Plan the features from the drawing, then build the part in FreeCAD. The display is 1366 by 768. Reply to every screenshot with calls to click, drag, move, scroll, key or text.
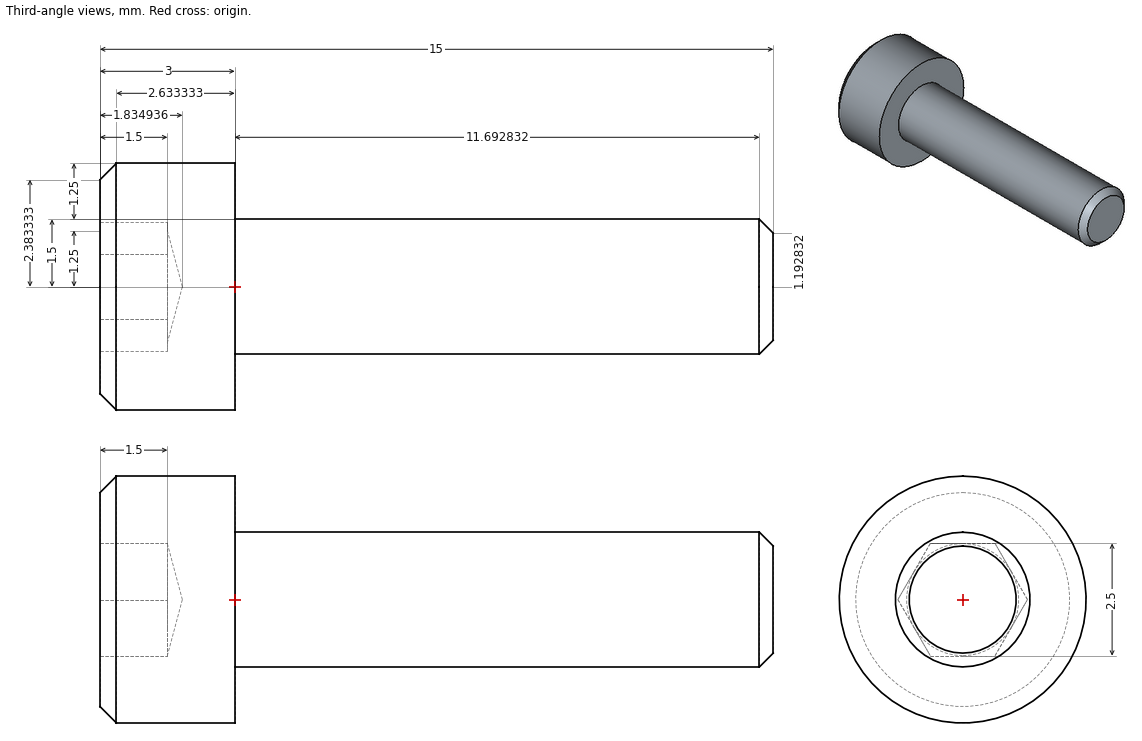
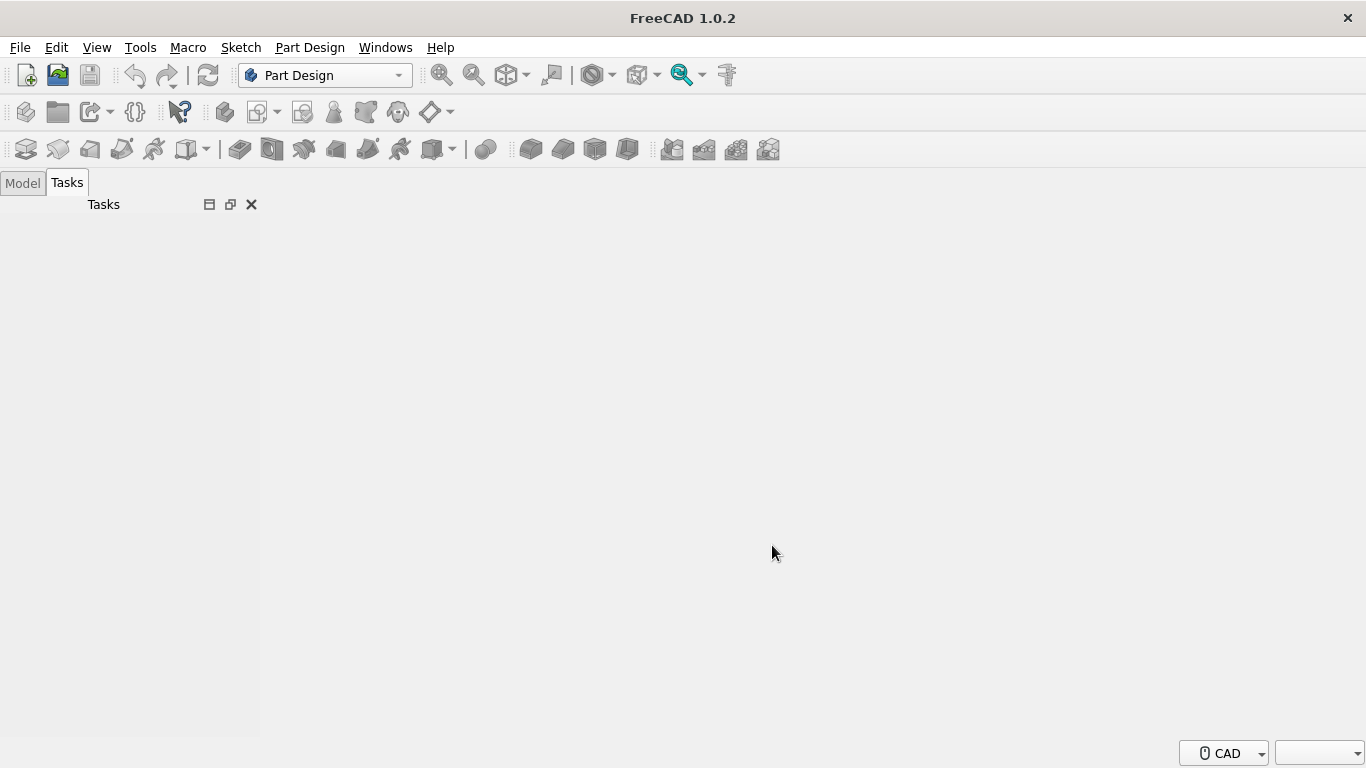
click(26, 76)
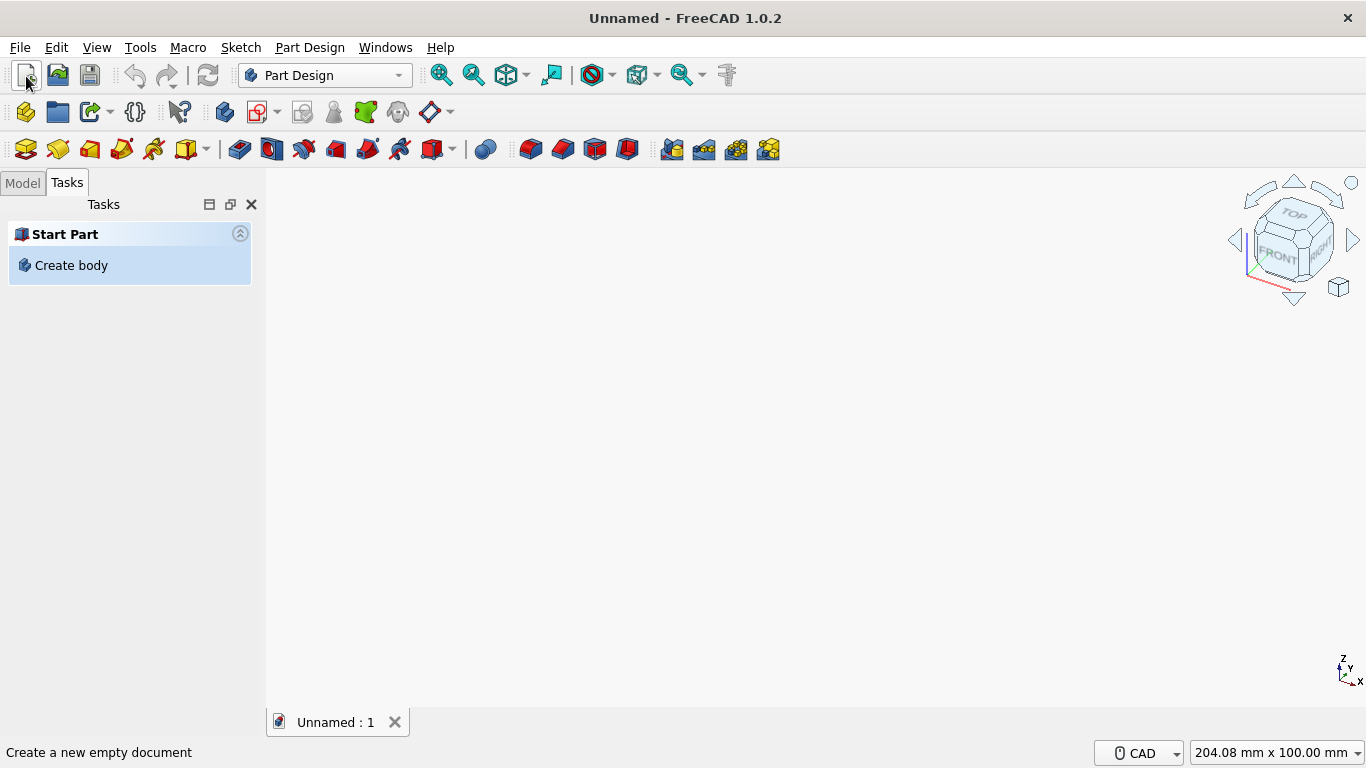
click(258, 112)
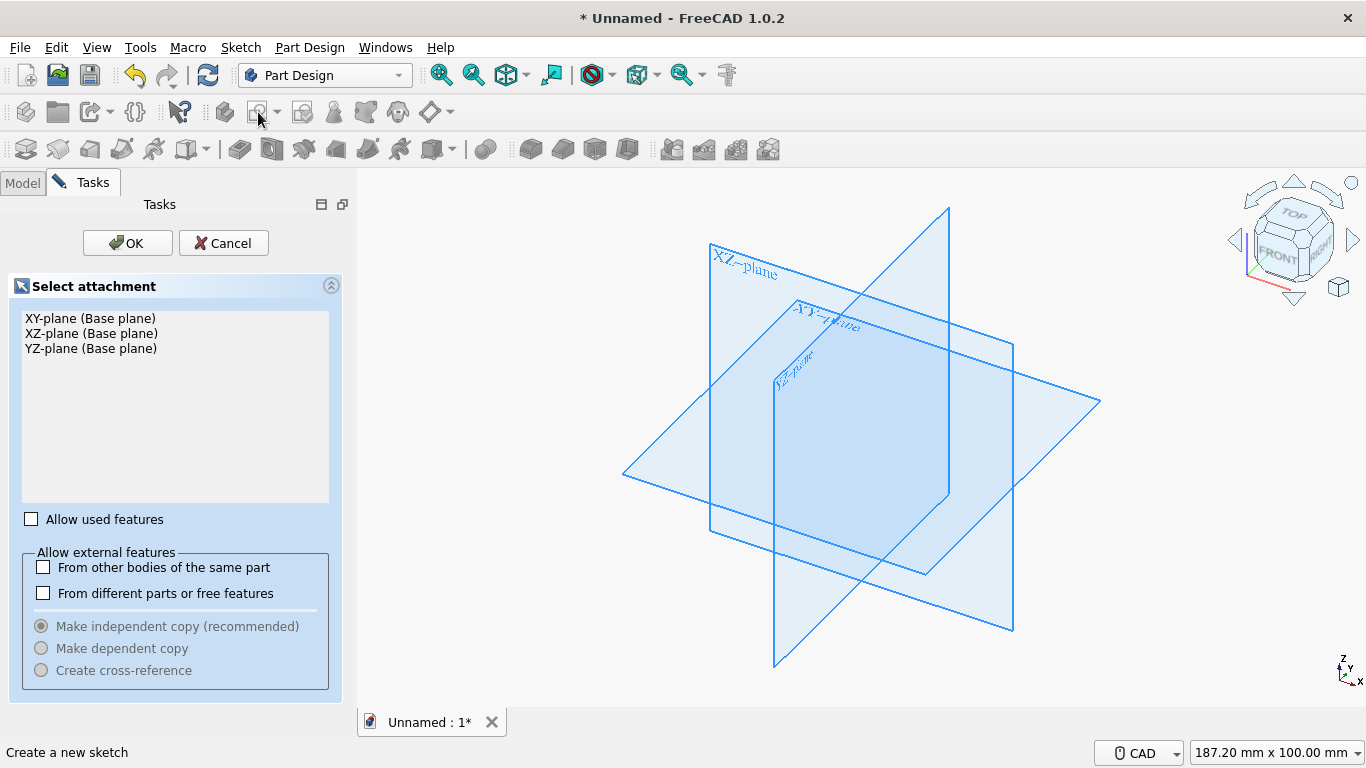
click(82, 318)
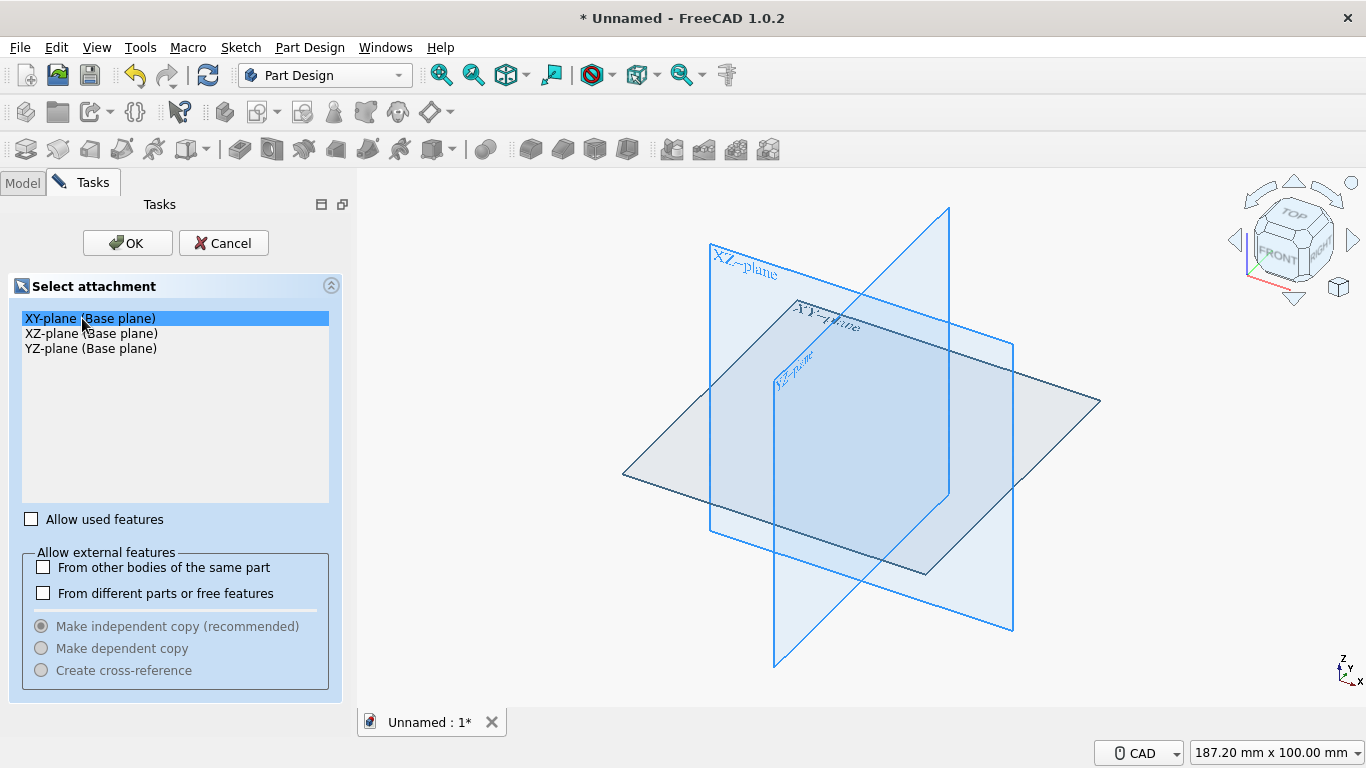
click(128, 243)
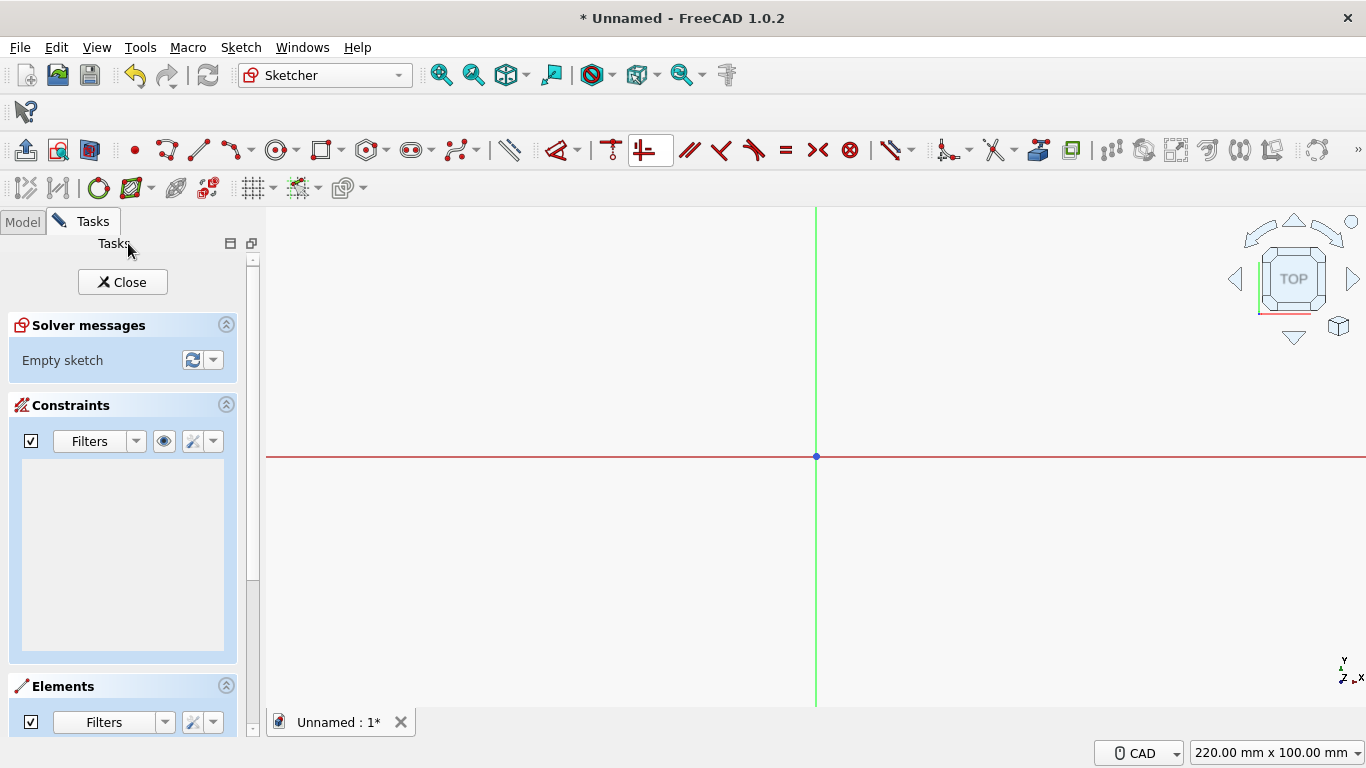
scroll(850, 449, up, 11)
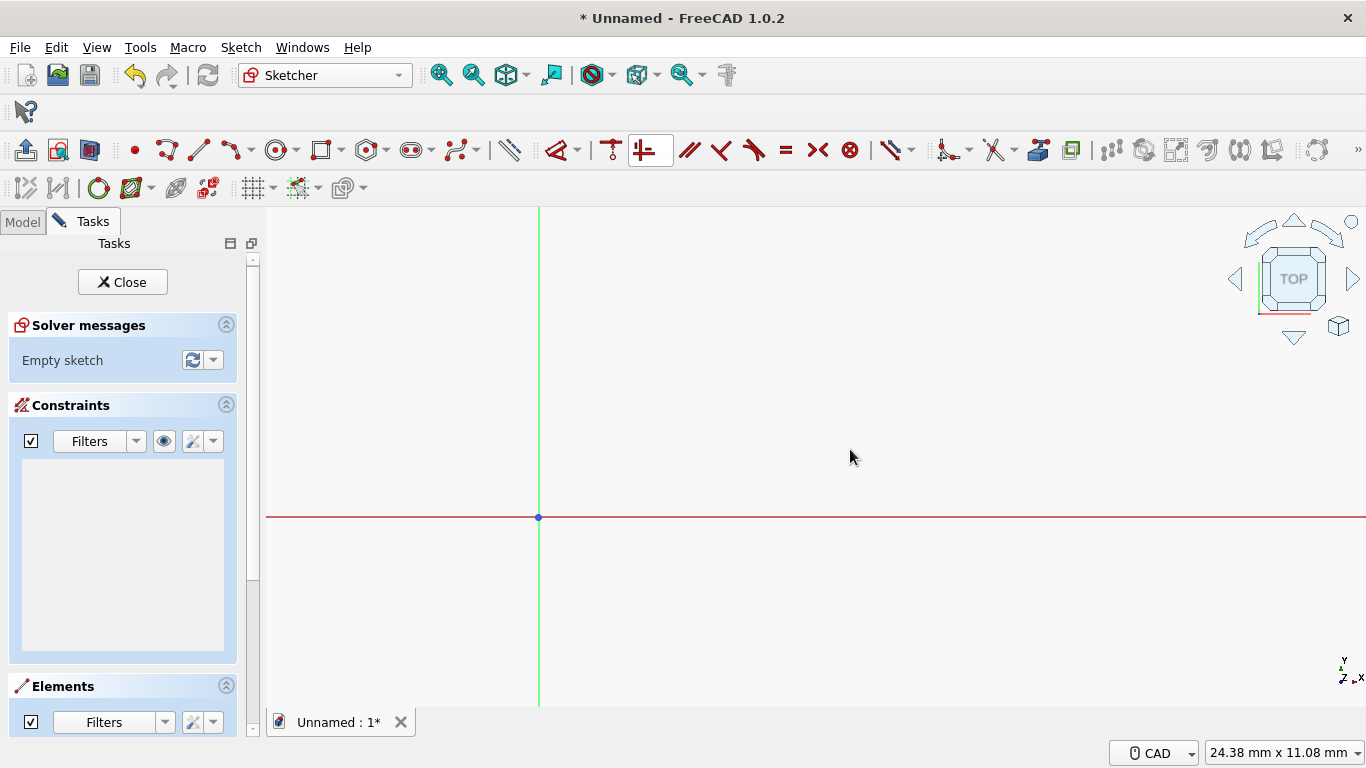
click(168, 150)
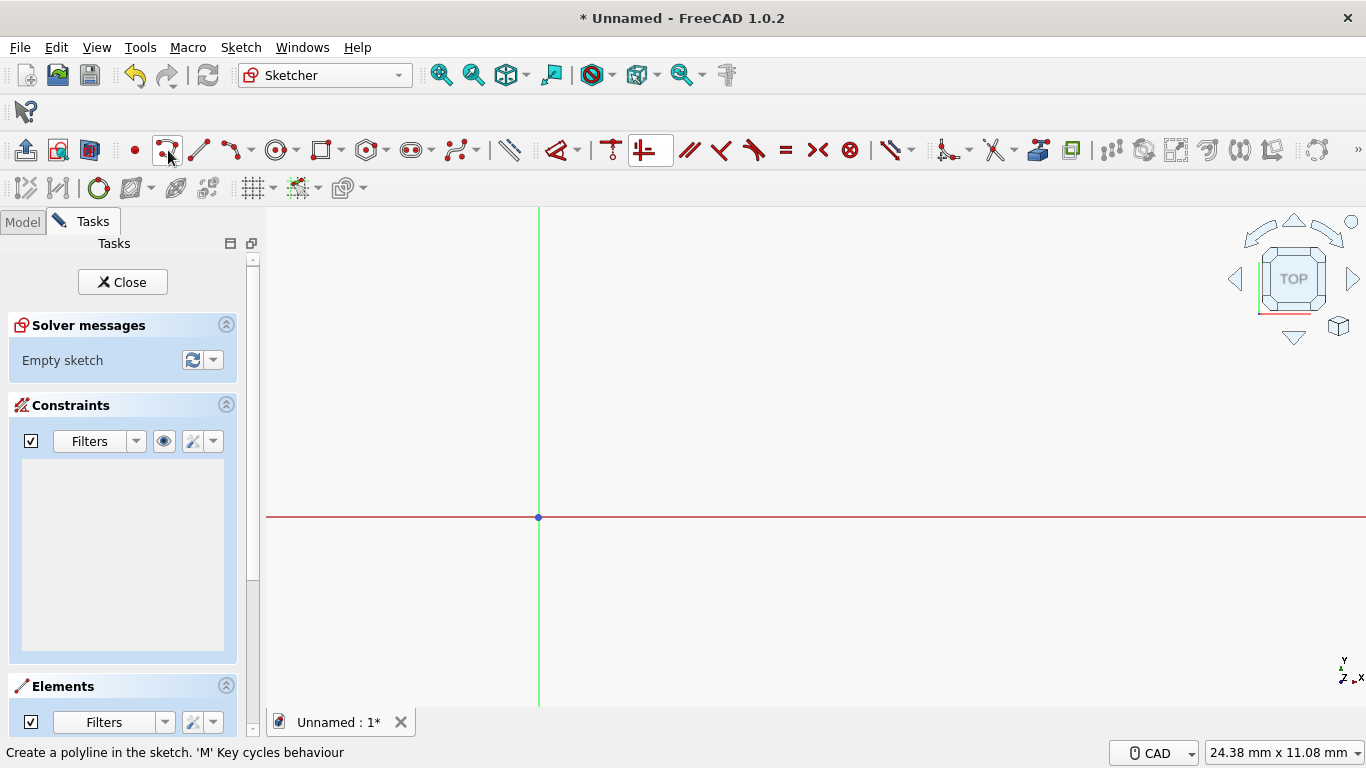
click(539, 450)
click(548, 393)
click(420, 393)
click(404, 410)
click(404, 517)
click(1080, 508)
click(1080, 463)
click(1067, 450)
click(539, 451)
key(Escape)
key(Escape)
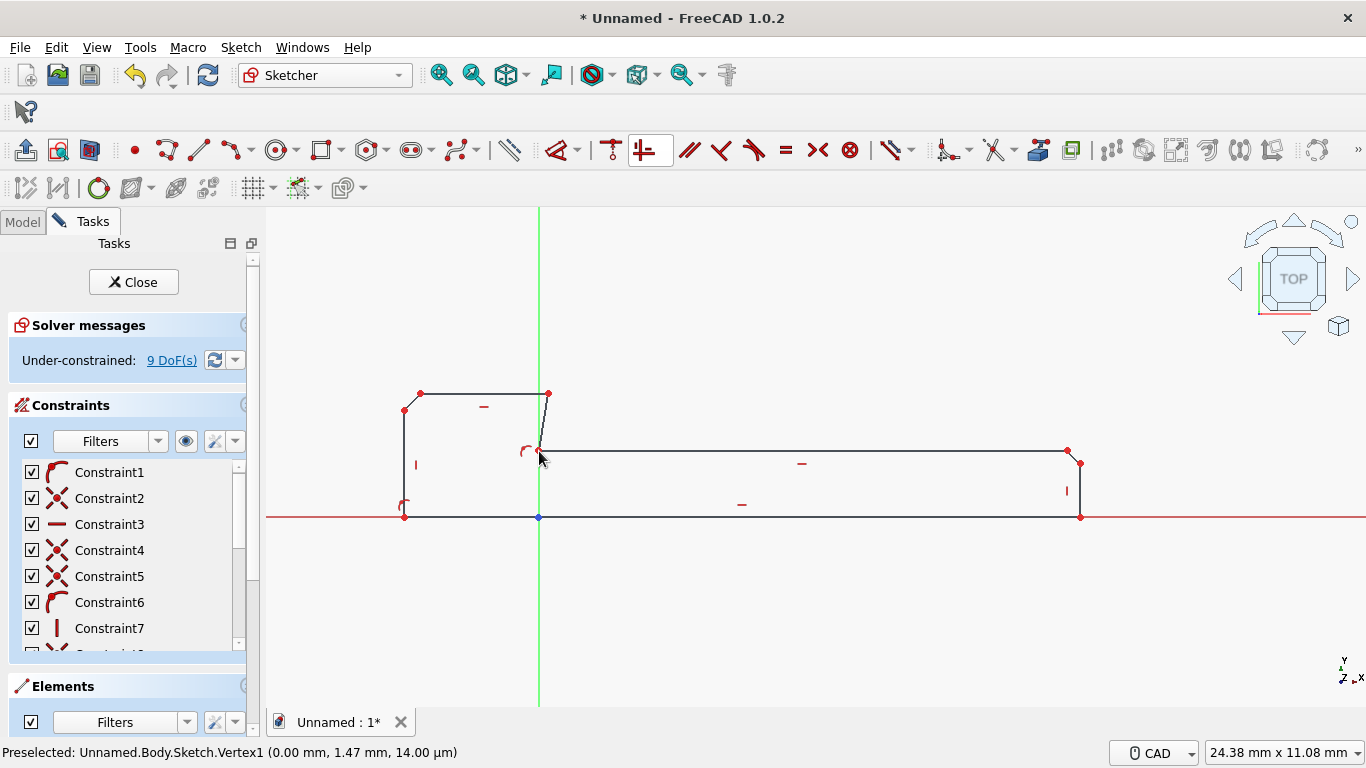
click(542, 434)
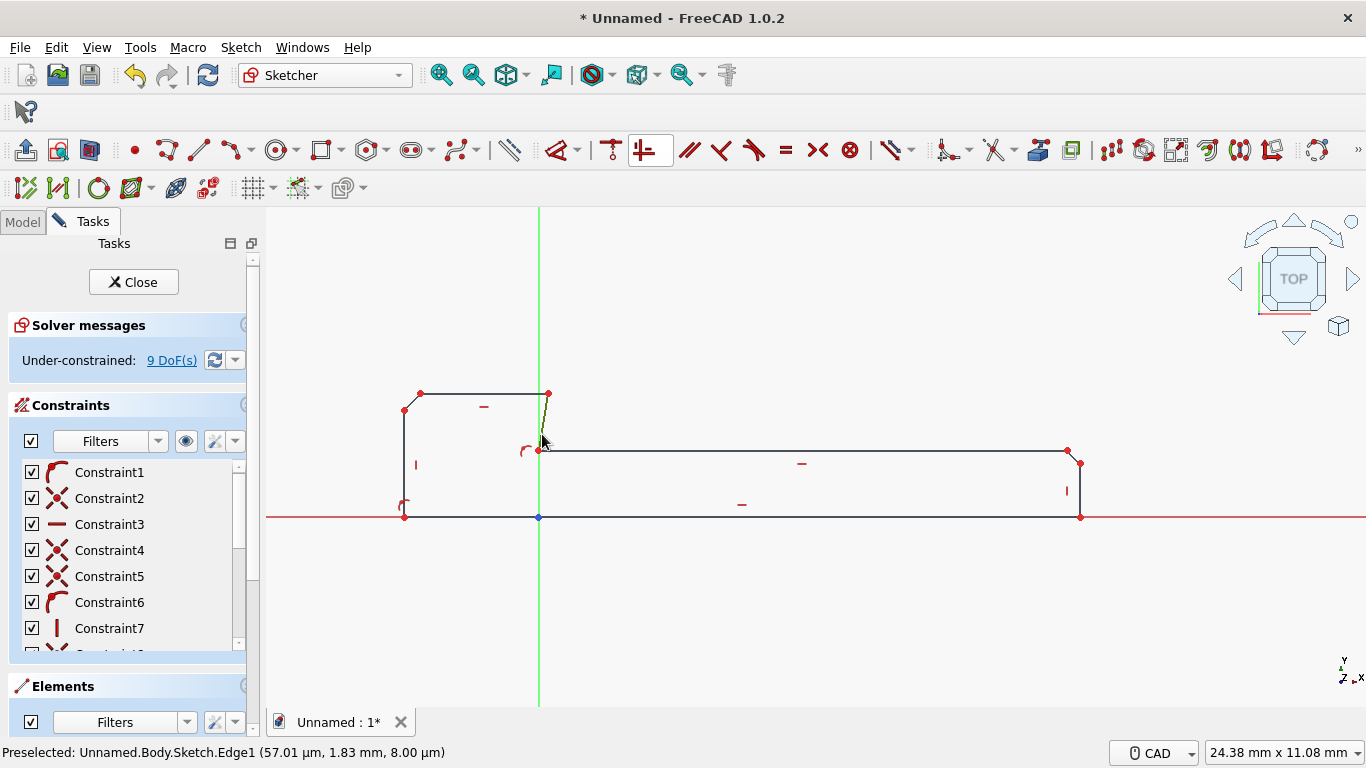
click(668, 150)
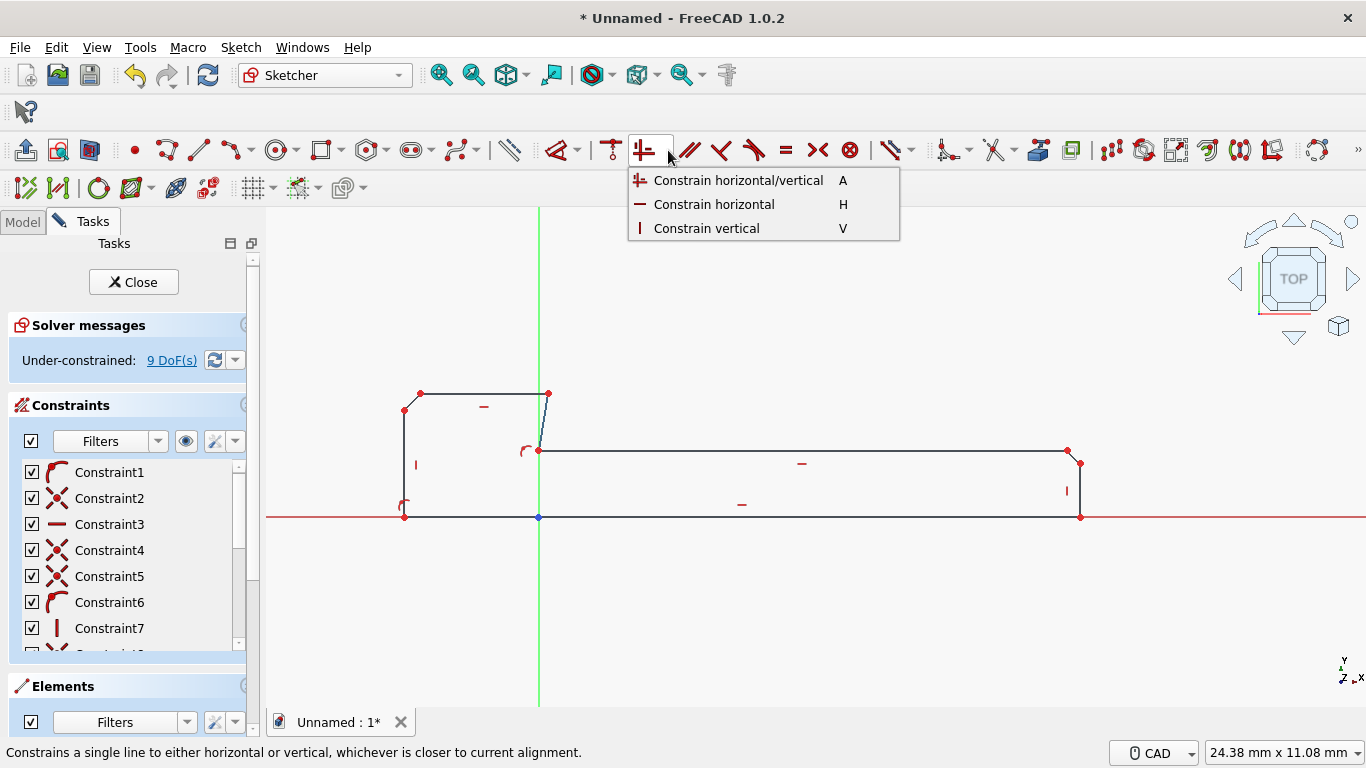
click(764, 228)